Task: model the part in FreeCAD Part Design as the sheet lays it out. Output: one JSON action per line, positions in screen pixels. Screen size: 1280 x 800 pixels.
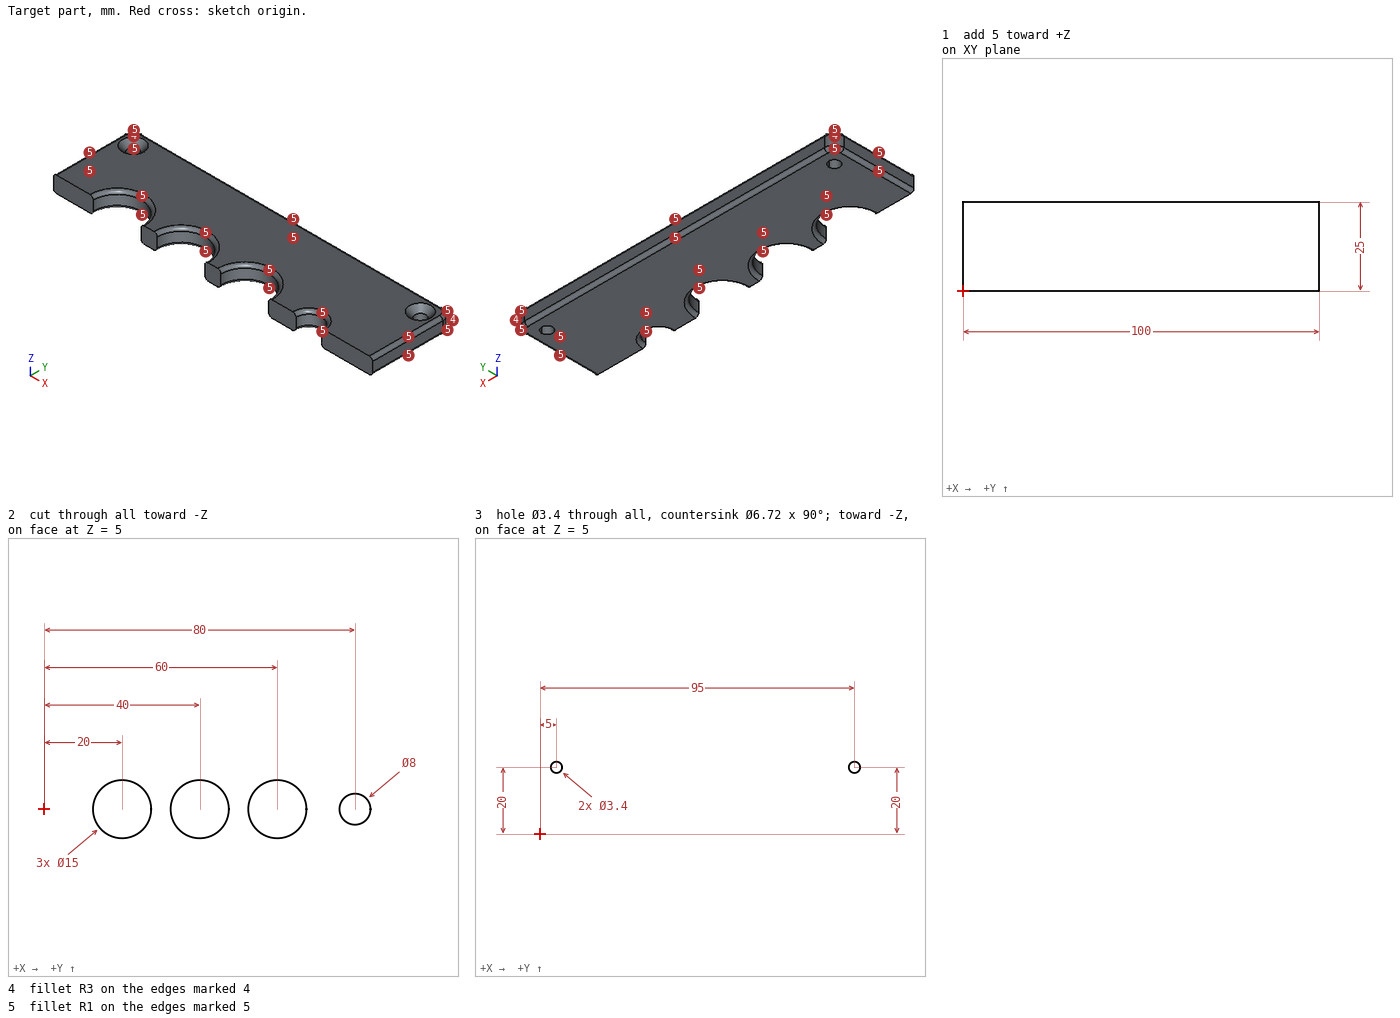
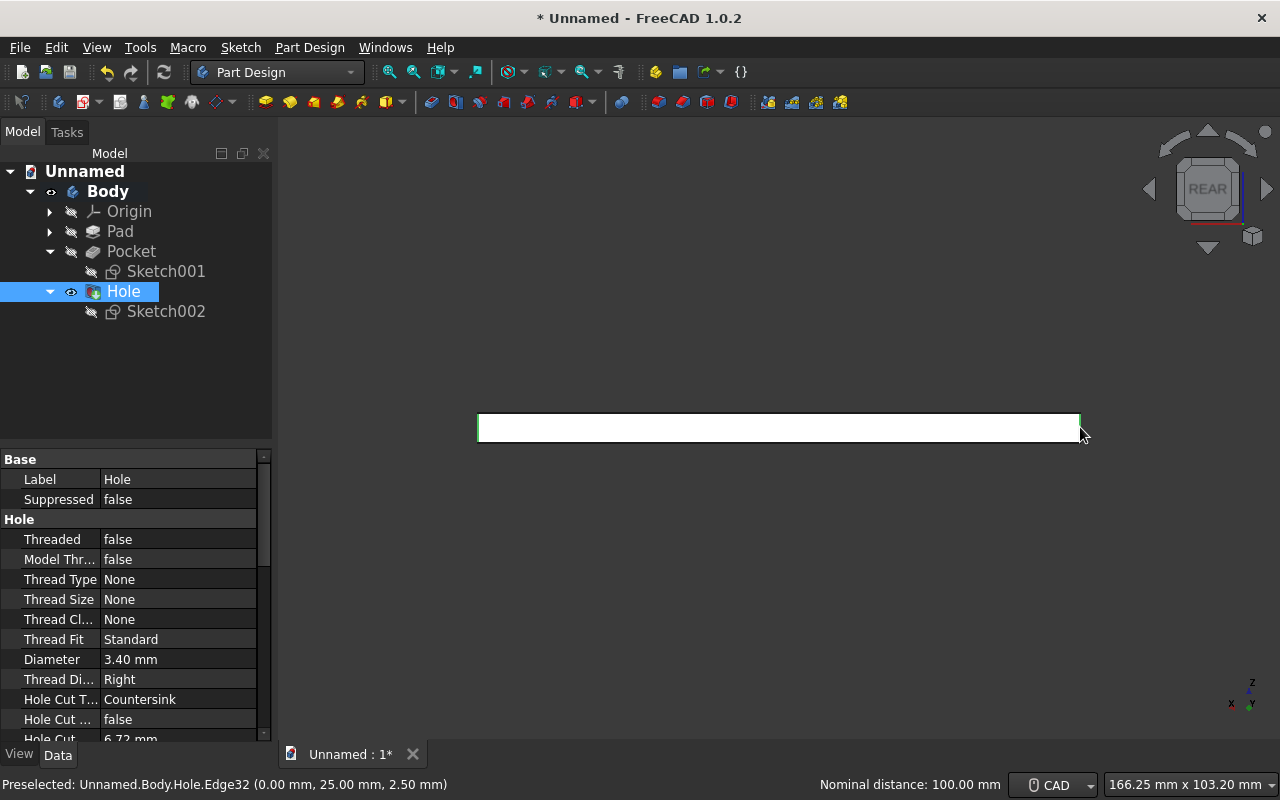
{"action": "left_click", "coordinate": [660, 102]}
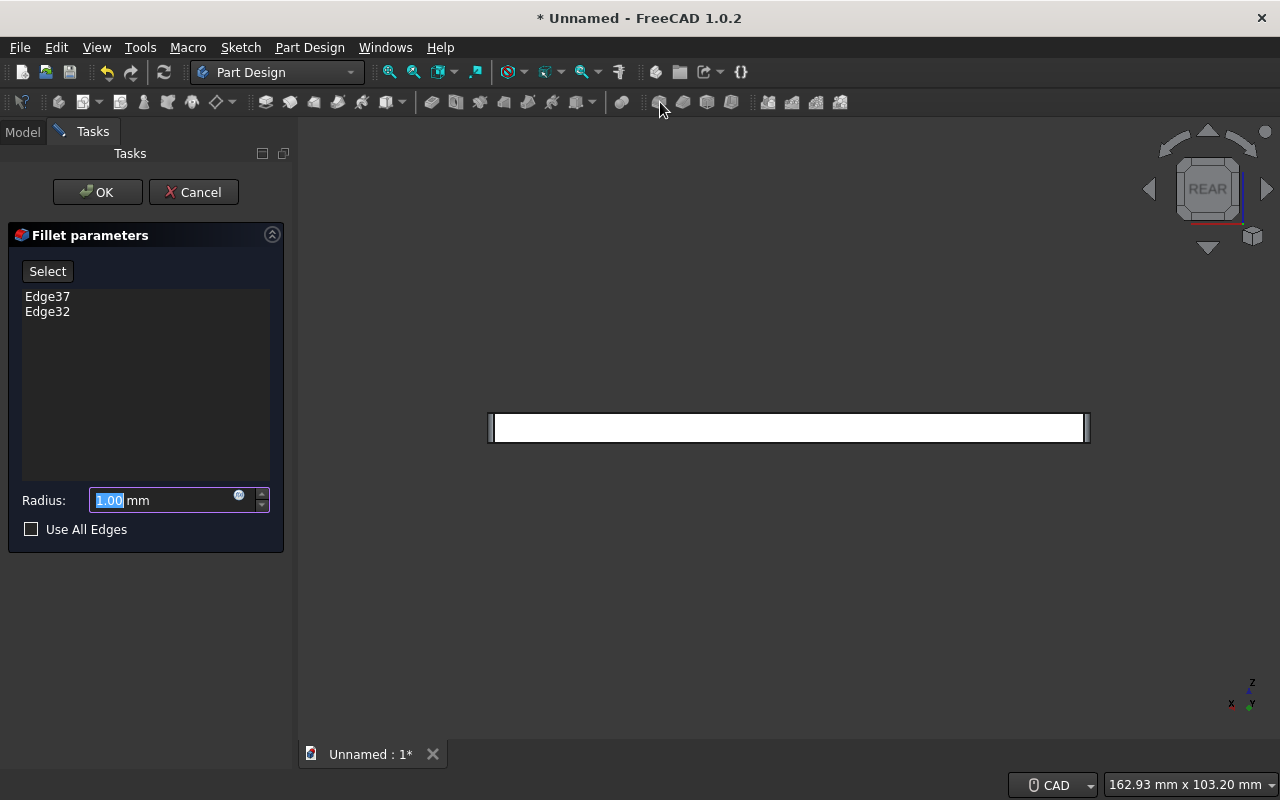
{"action": "type", "text": "3"}
{"action": "key", "text": "Tab"}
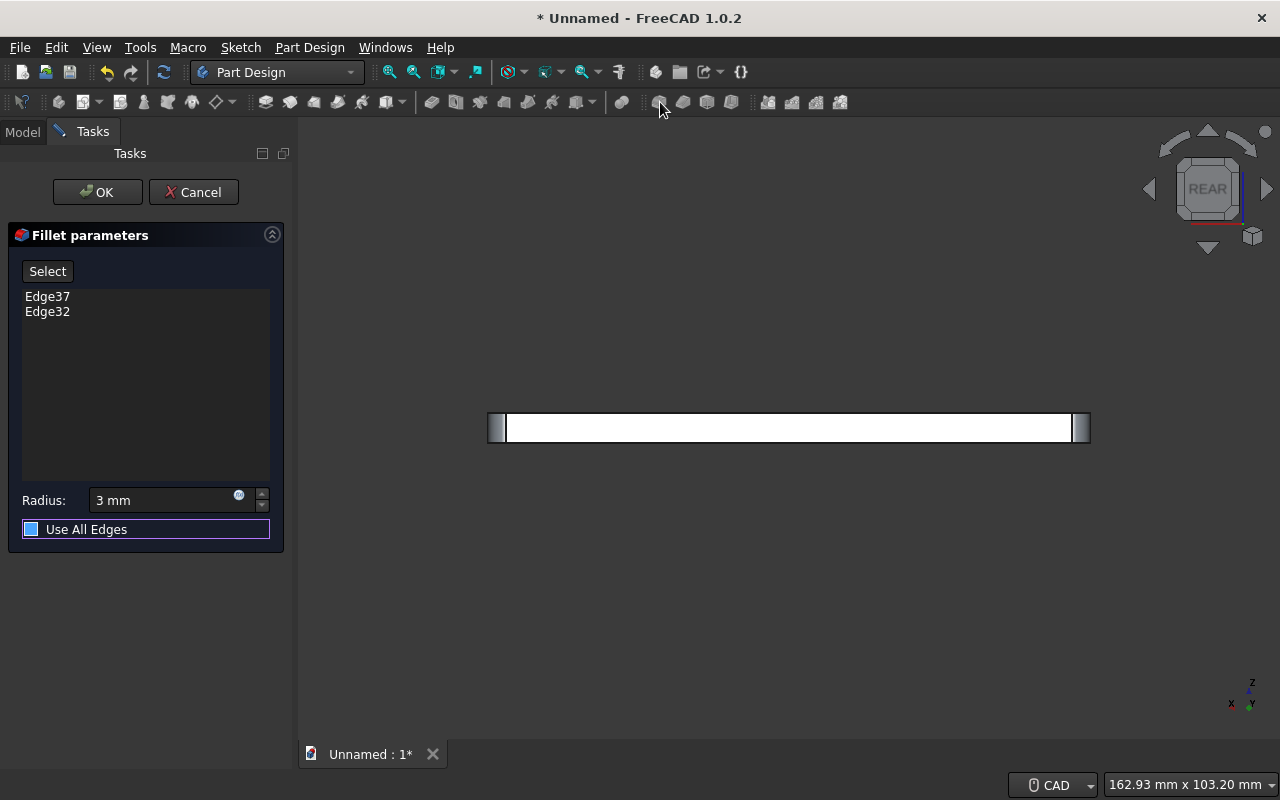
{"action": "left_click", "coordinate": [98, 192]}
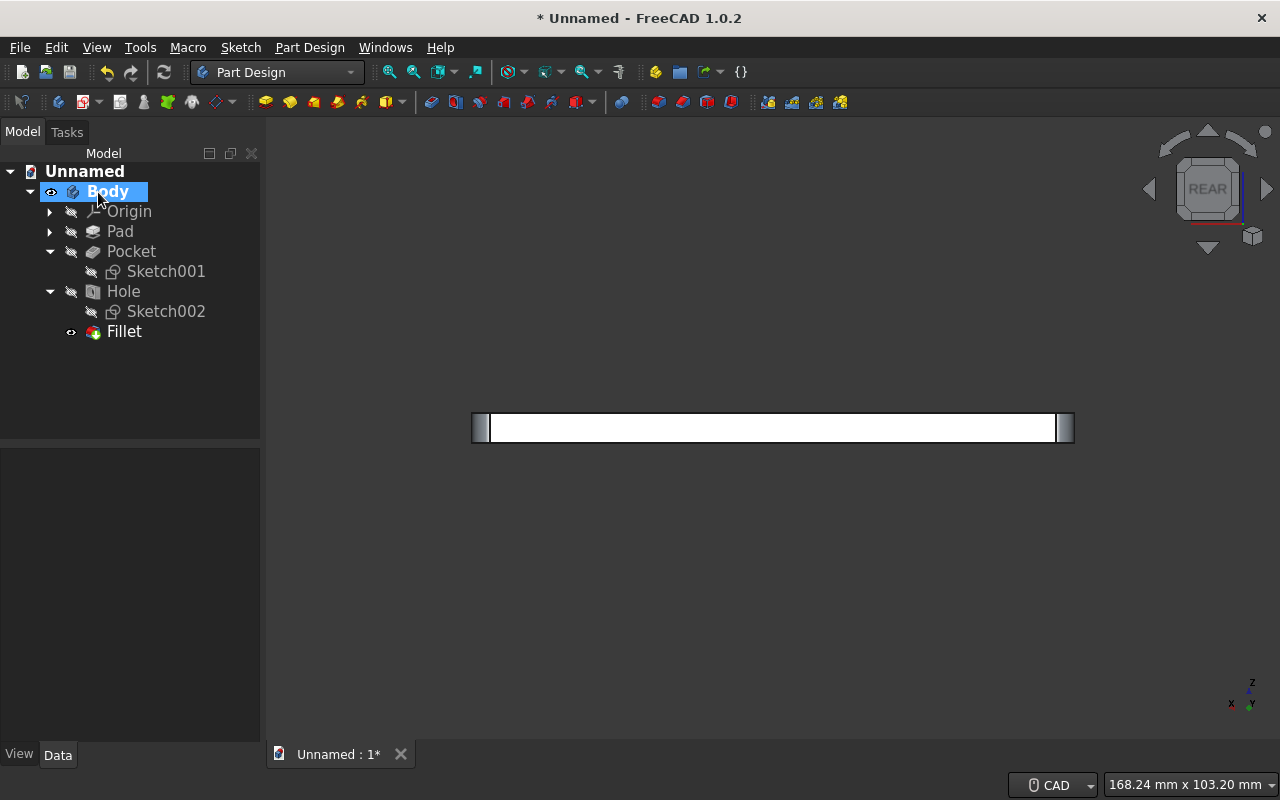
{"action": "left_click", "coordinate": [773, 442]}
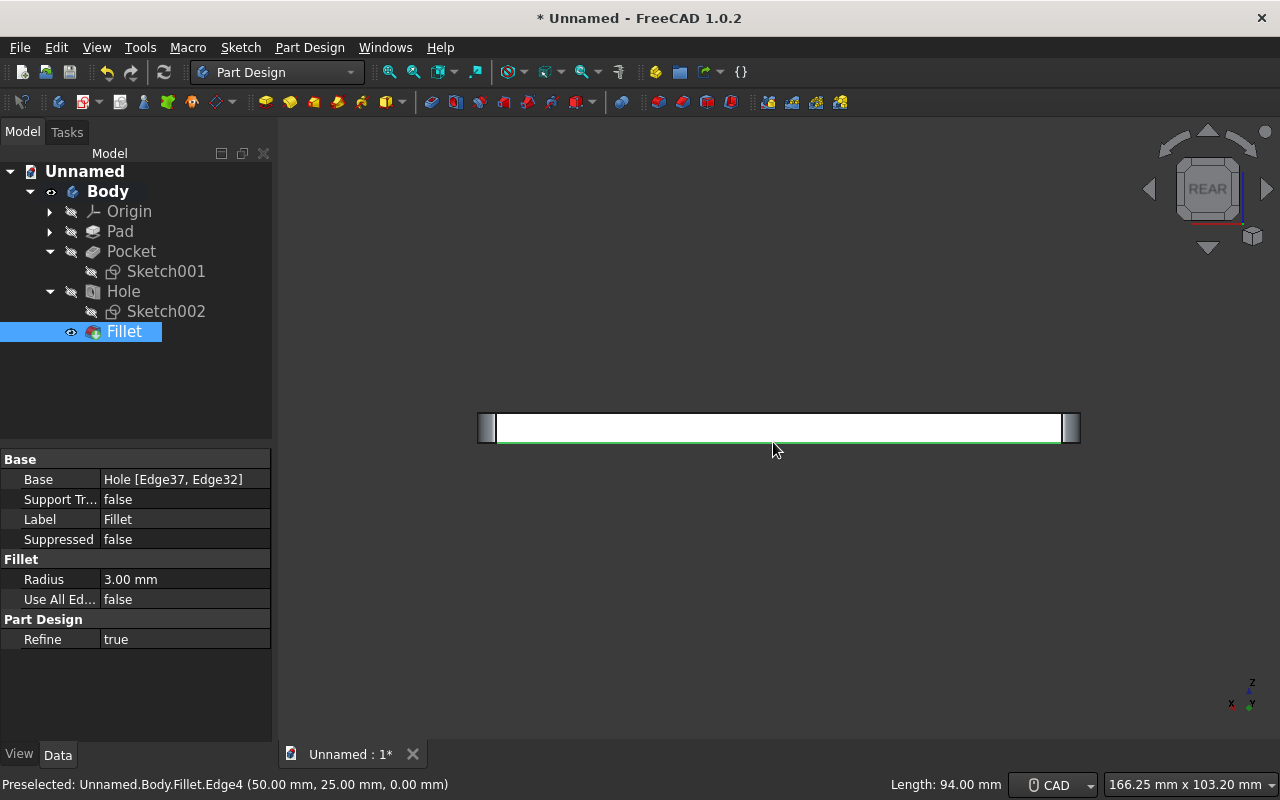
{"action": "left_click", "coordinate": [779, 412], "text": "ctrl"}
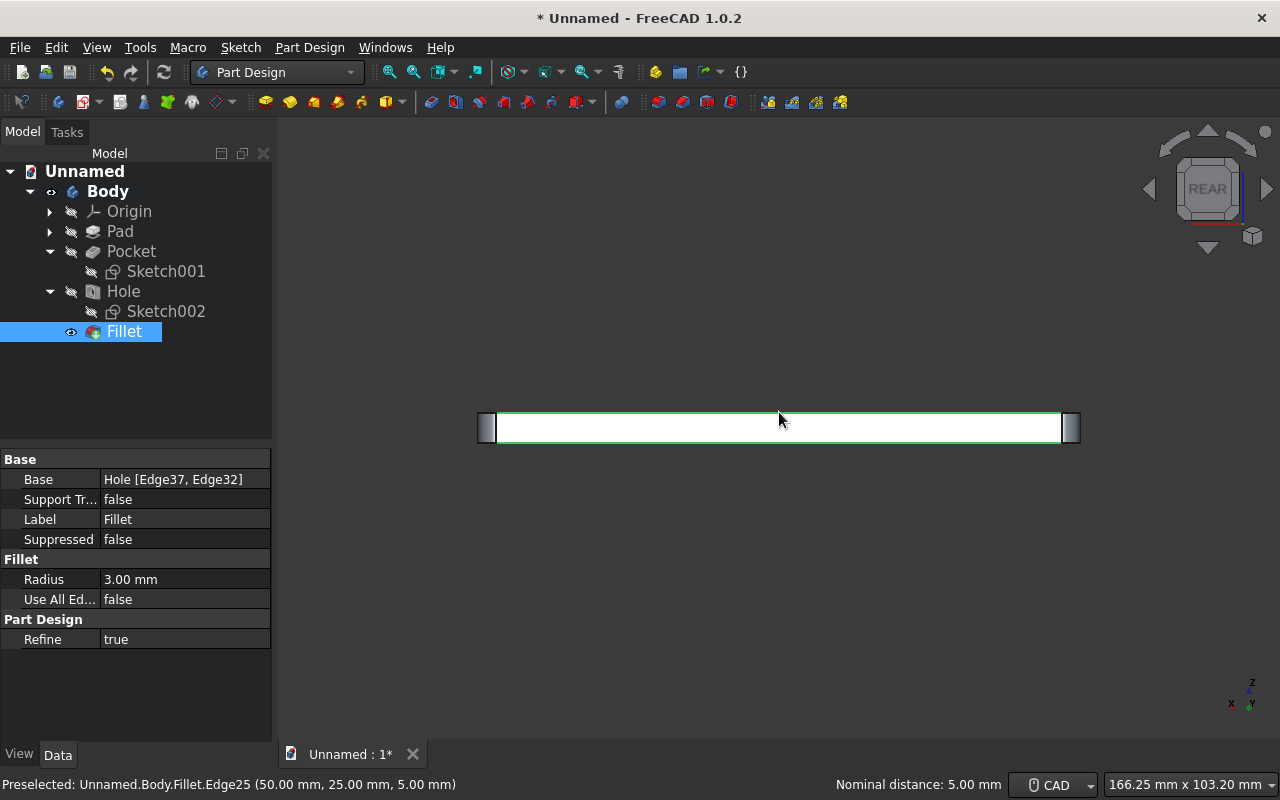
{"action": "left_click", "coordinate": [1075, 442], "text": "ctrl"}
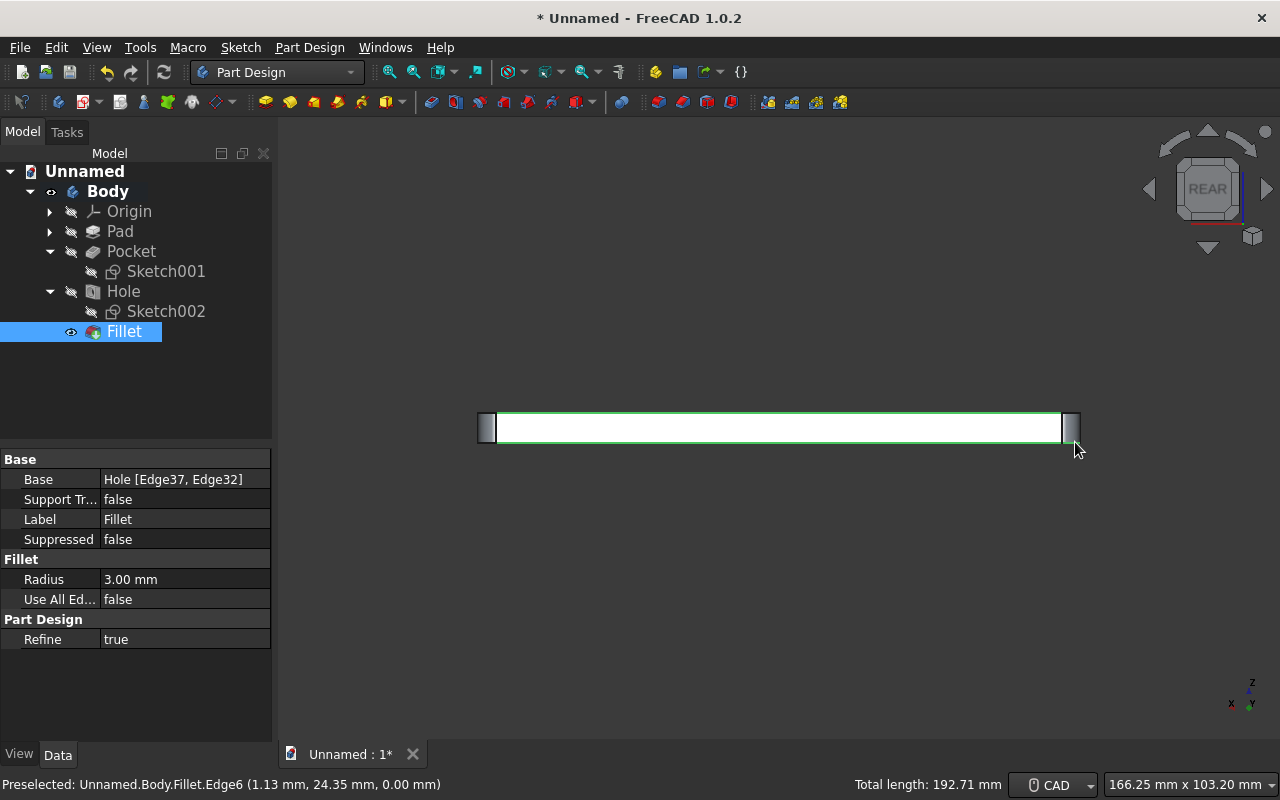
{"action": "left_click", "coordinate": [483, 442], "text": "ctrl"}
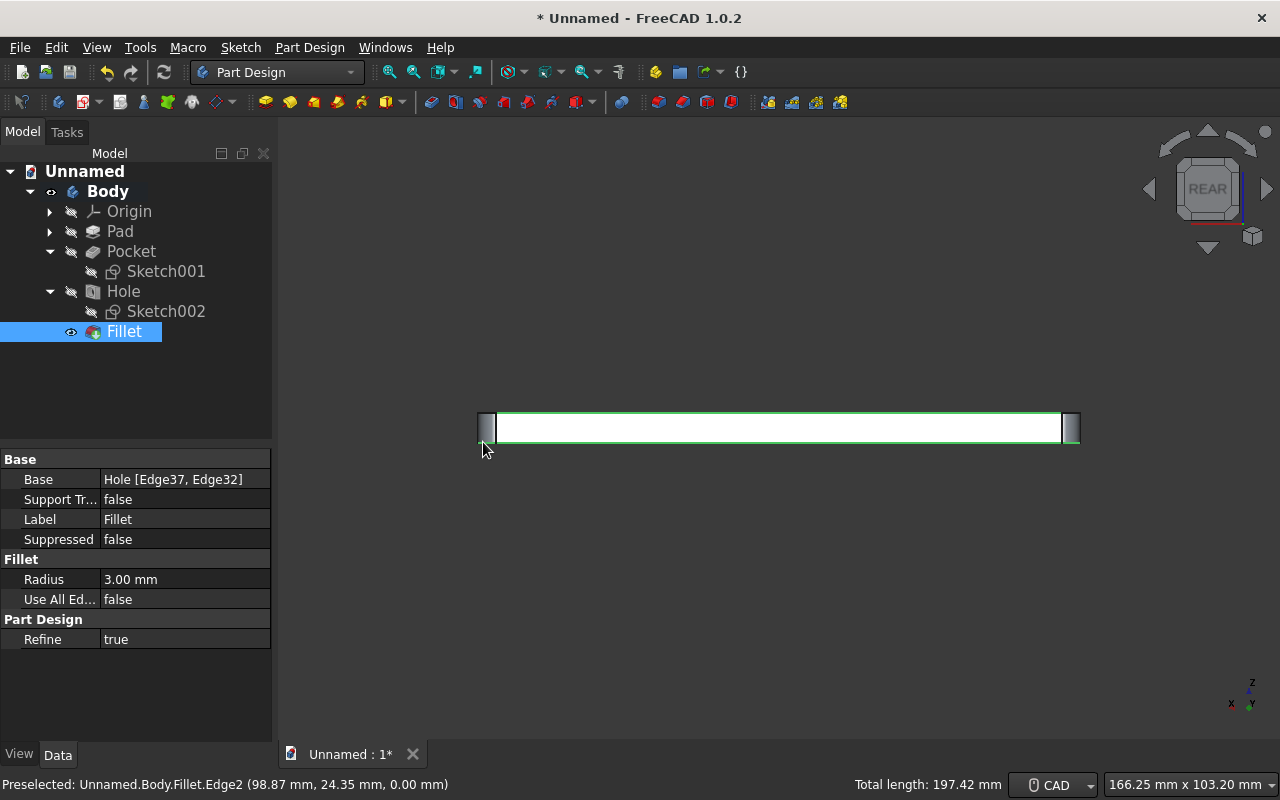
{"action": "left_click", "coordinate": [1075, 412], "text": "ctrl"}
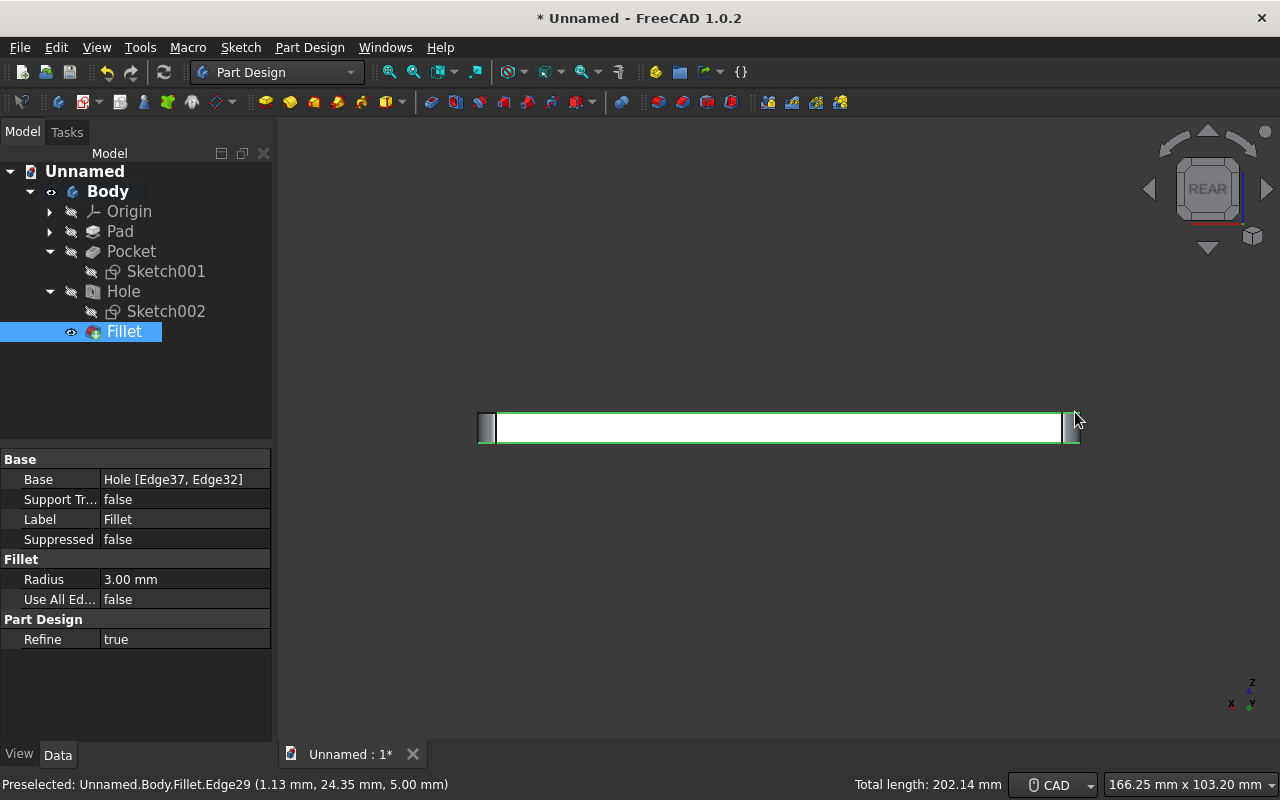
{"action": "left_click", "coordinate": [483, 412], "text": "ctrl"}